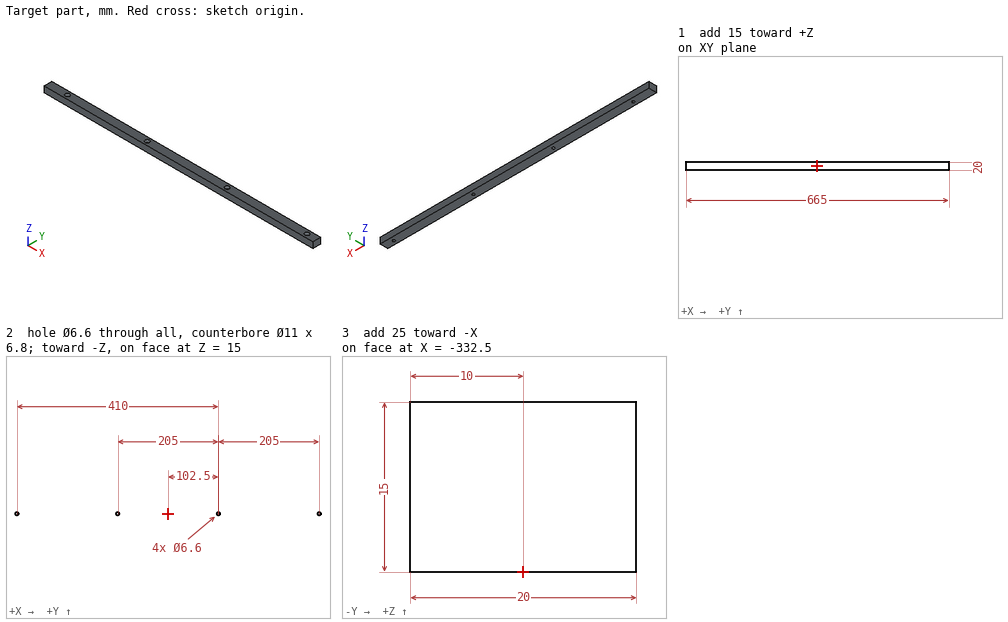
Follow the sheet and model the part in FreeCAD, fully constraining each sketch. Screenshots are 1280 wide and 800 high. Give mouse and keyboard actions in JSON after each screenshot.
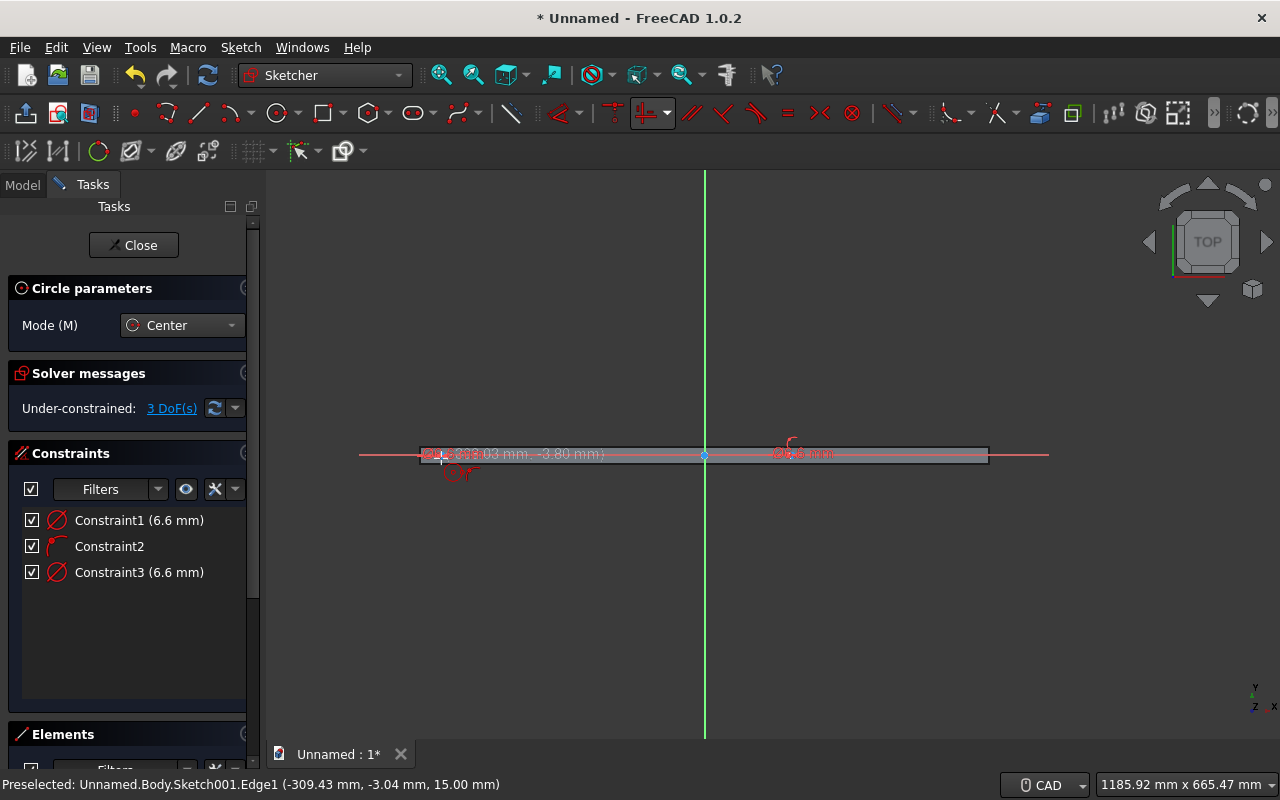
{"action": "scroll", "coordinate": [967, 455], "scroll_direction": "up", "scroll_amount": 11}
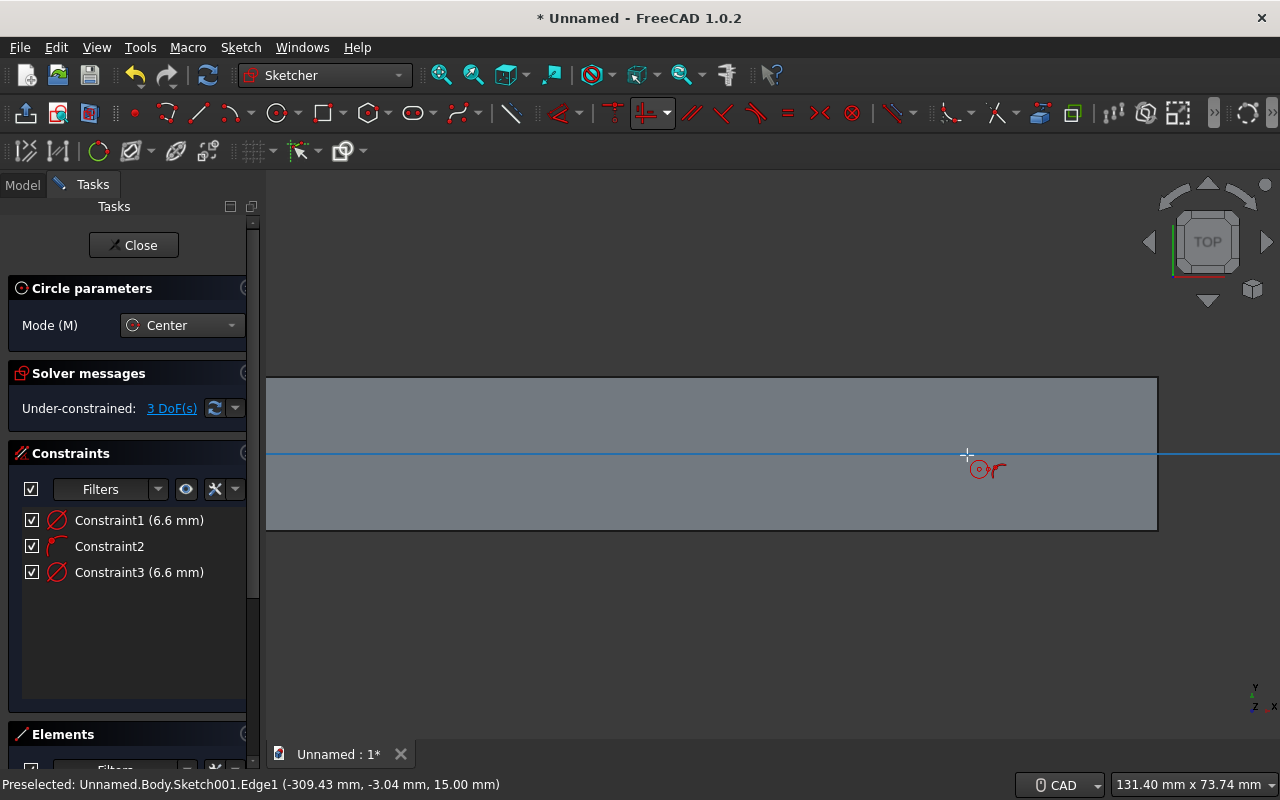
{"action": "scroll", "coordinate": [968, 455], "scroll_direction": "down", "scroll_amount": 11}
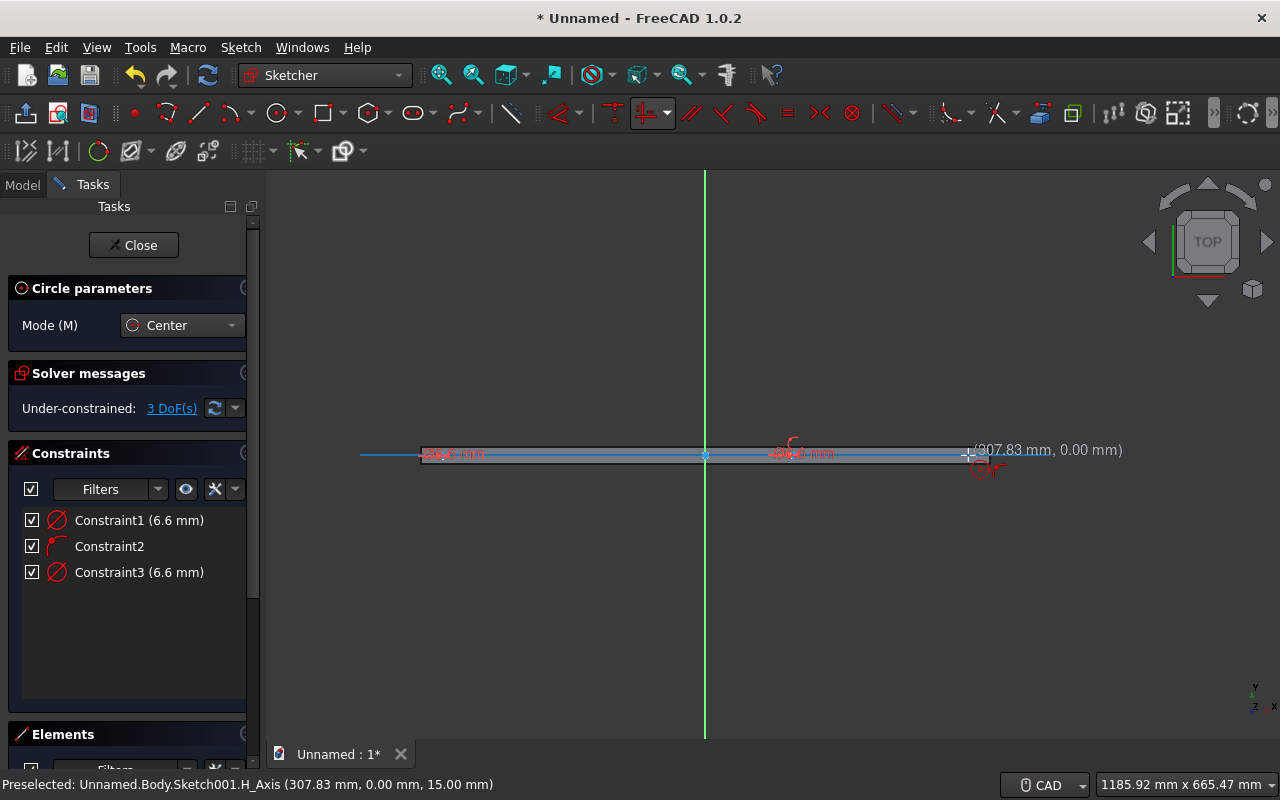
{"action": "left_click", "coordinate": [968, 455]}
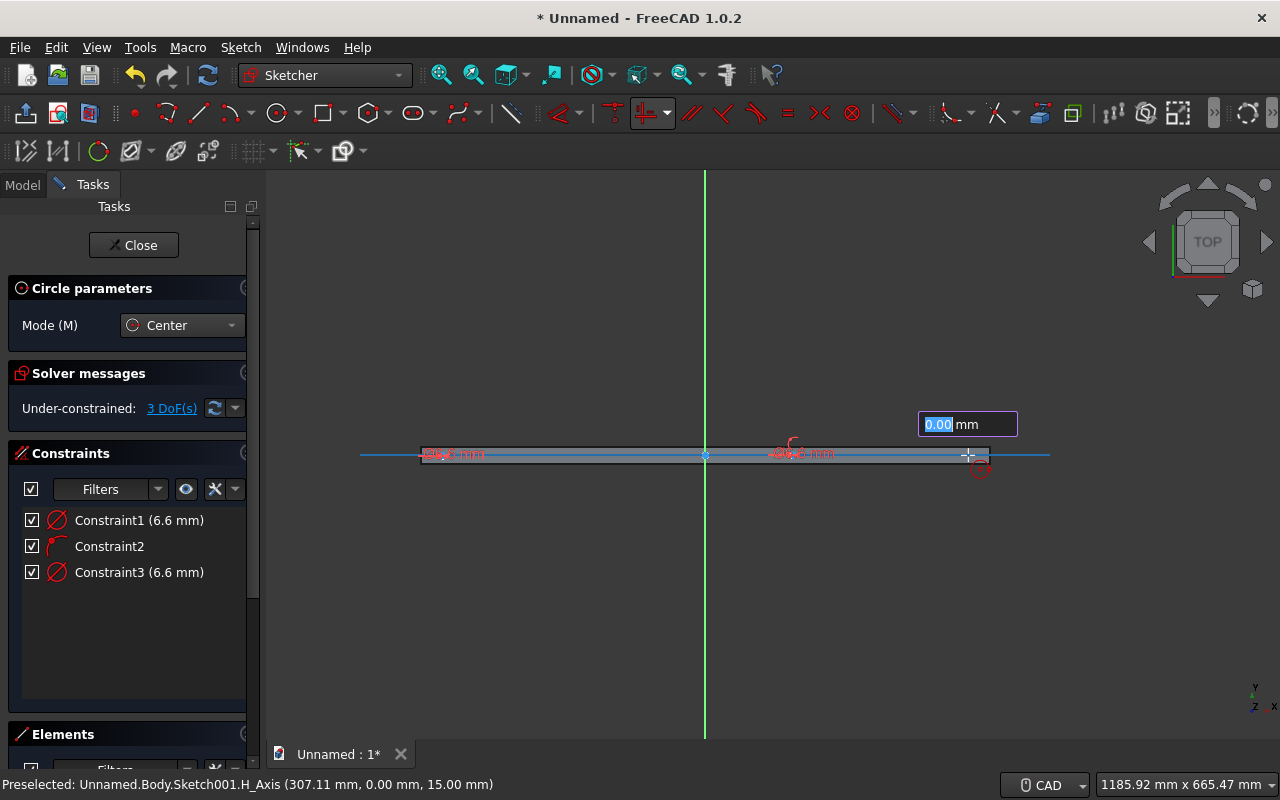
{"action": "scroll", "coordinate": [969, 453], "scroll_direction": "up", "scroll_amount": 9}
{"action": "mouse_move", "coordinate": [967, 449]}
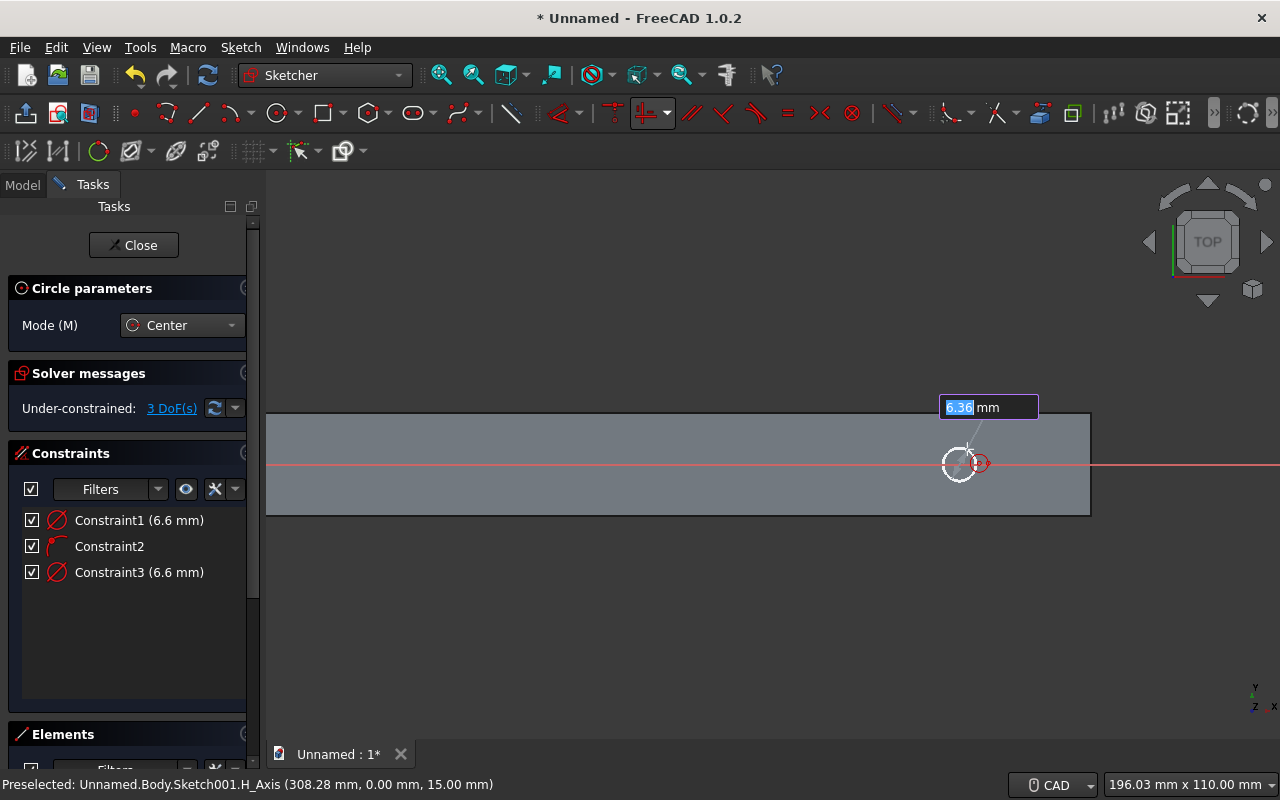
{"action": "type", "text": "6.6"}
{"action": "key", "text": "Return"}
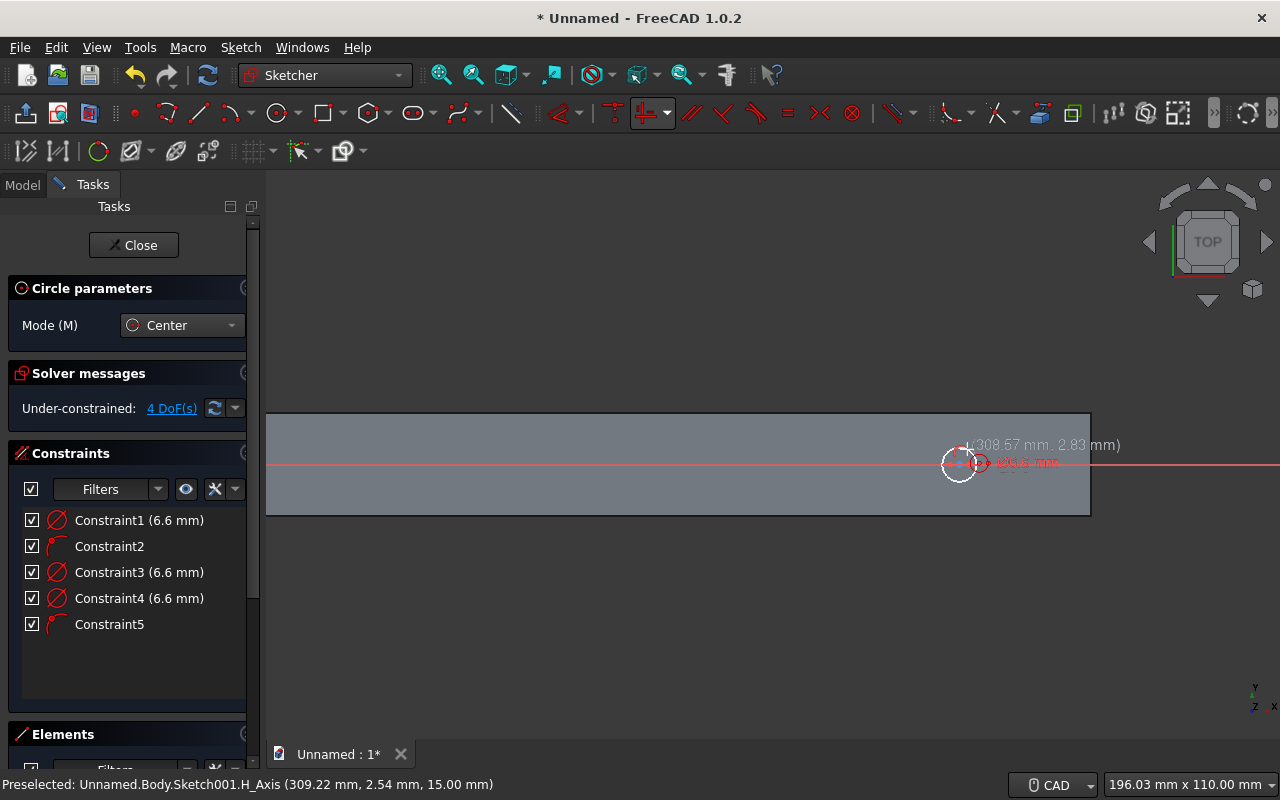
{"action": "scroll", "coordinate": [969, 452], "scroll_direction": "down", "scroll_amount": 9}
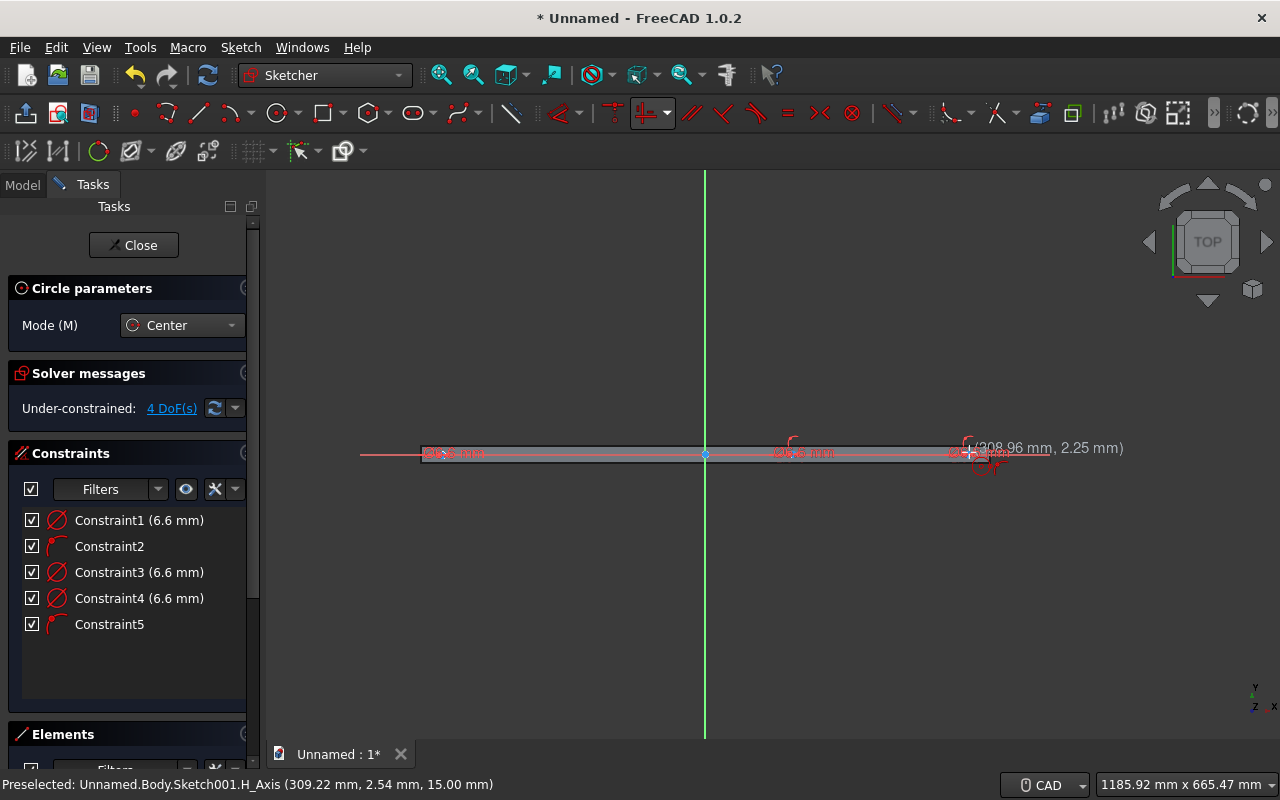
{"action": "scroll", "coordinate": [618, 454], "scroll_direction": "up", "scroll_amount": 11}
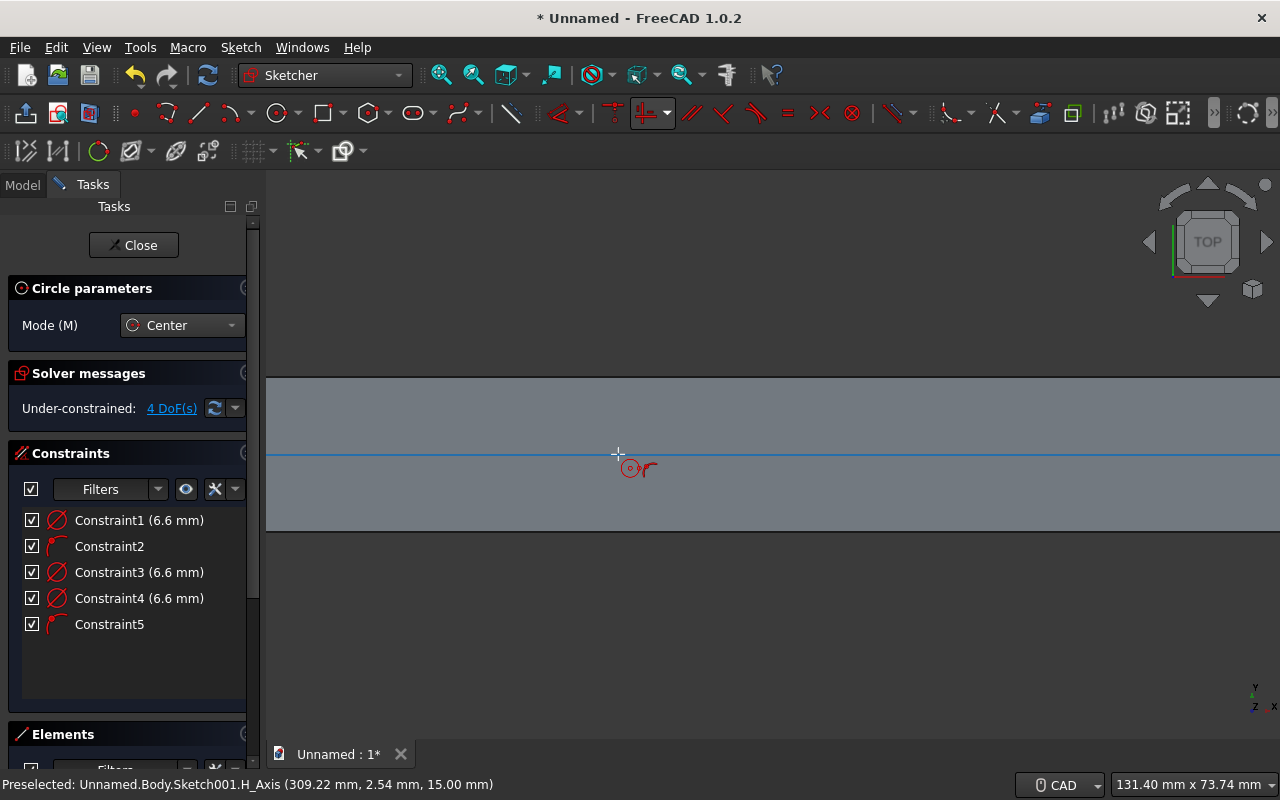
{"action": "scroll", "coordinate": [617, 455], "scroll_direction": "down", "scroll_amount": 11}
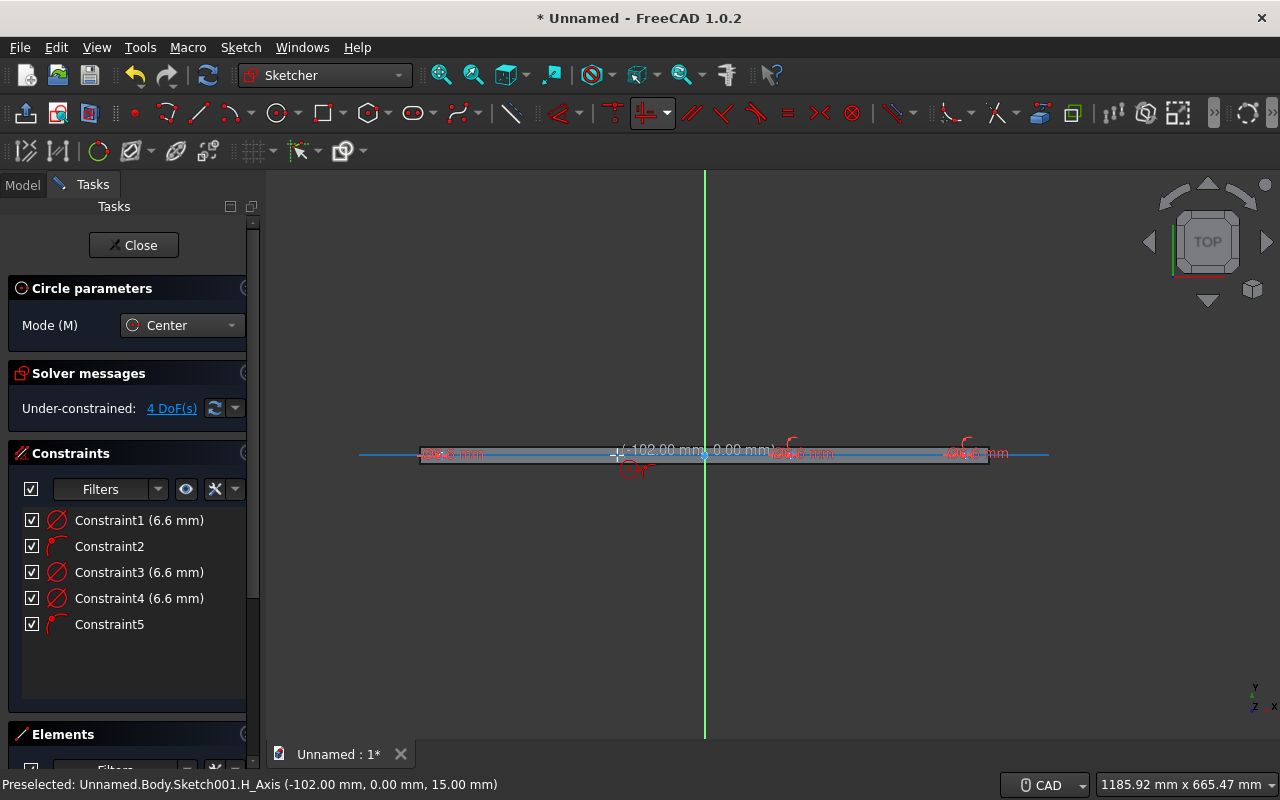
{"action": "left_click", "coordinate": [617, 455]}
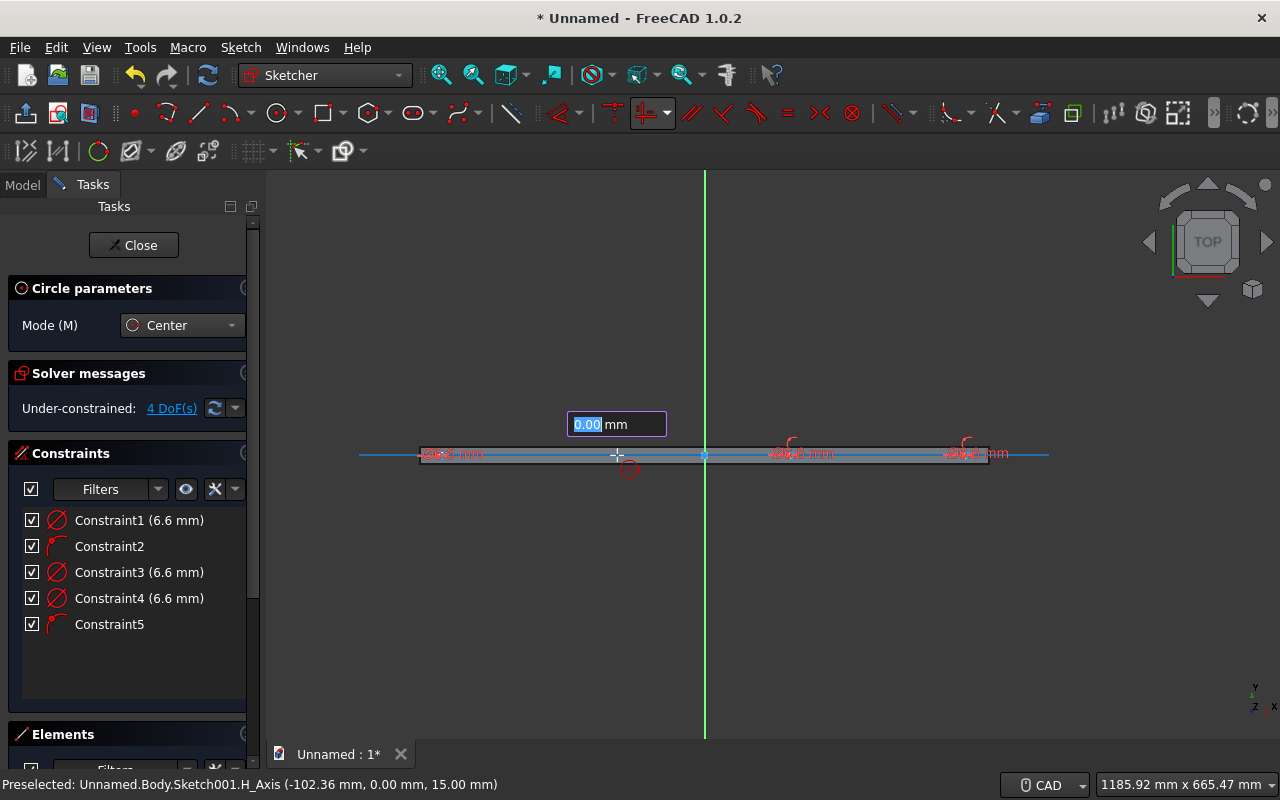
{"action": "scroll", "coordinate": [616, 458], "scroll_direction": "up", "scroll_amount": 9}
{"action": "mouse_move", "coordinate": [614, 456]}